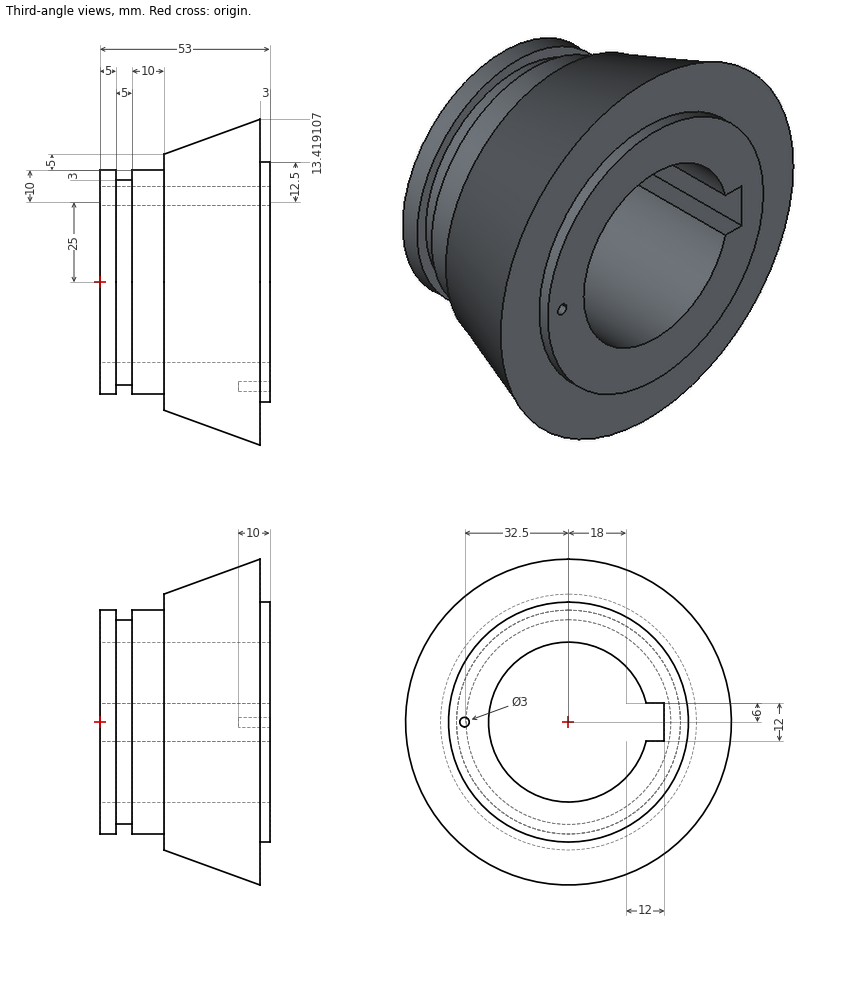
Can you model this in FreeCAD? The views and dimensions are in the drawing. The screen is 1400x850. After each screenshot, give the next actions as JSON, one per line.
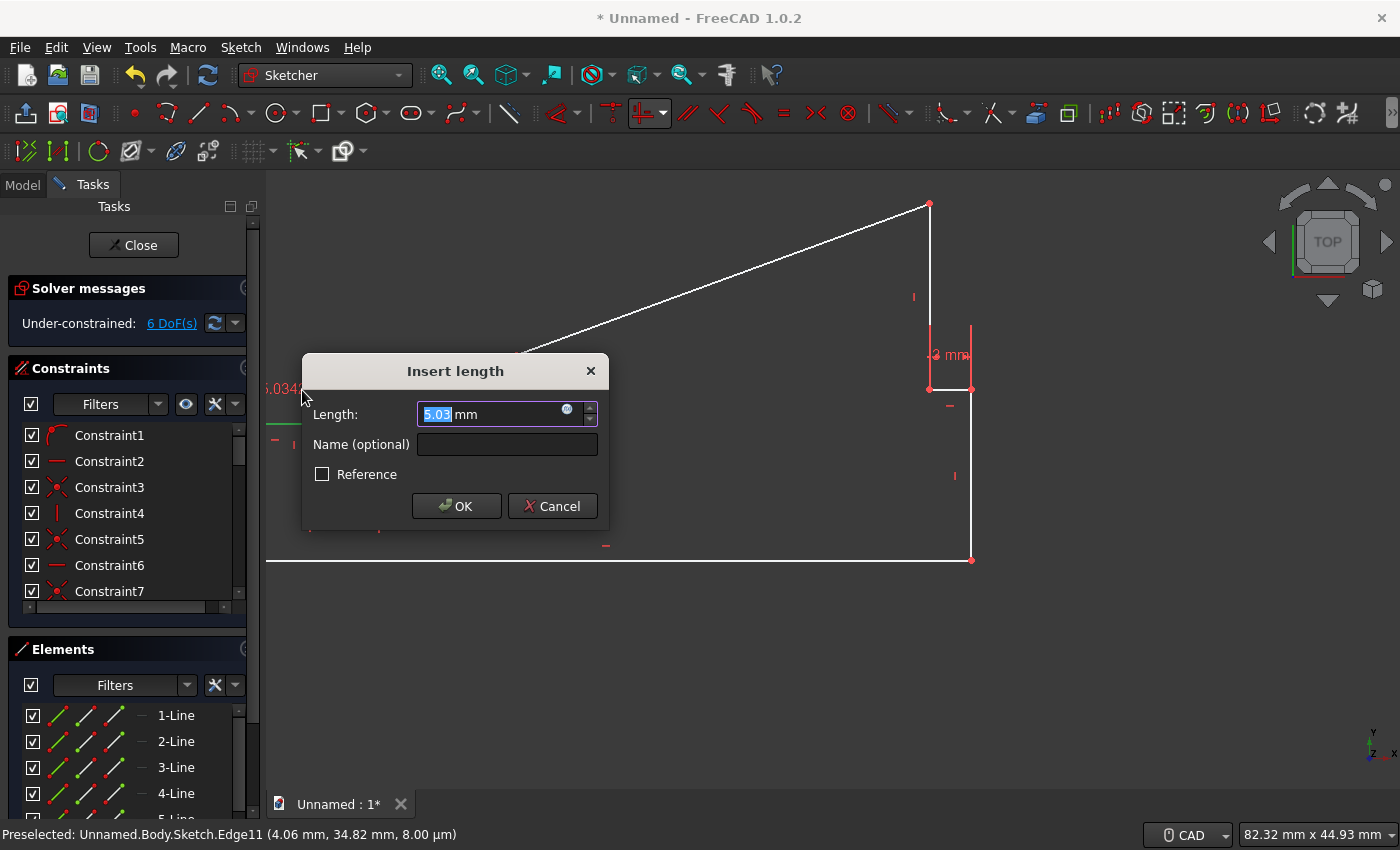
{"action": "type", "text": "5"}
{"action": "key", "text": "Return"}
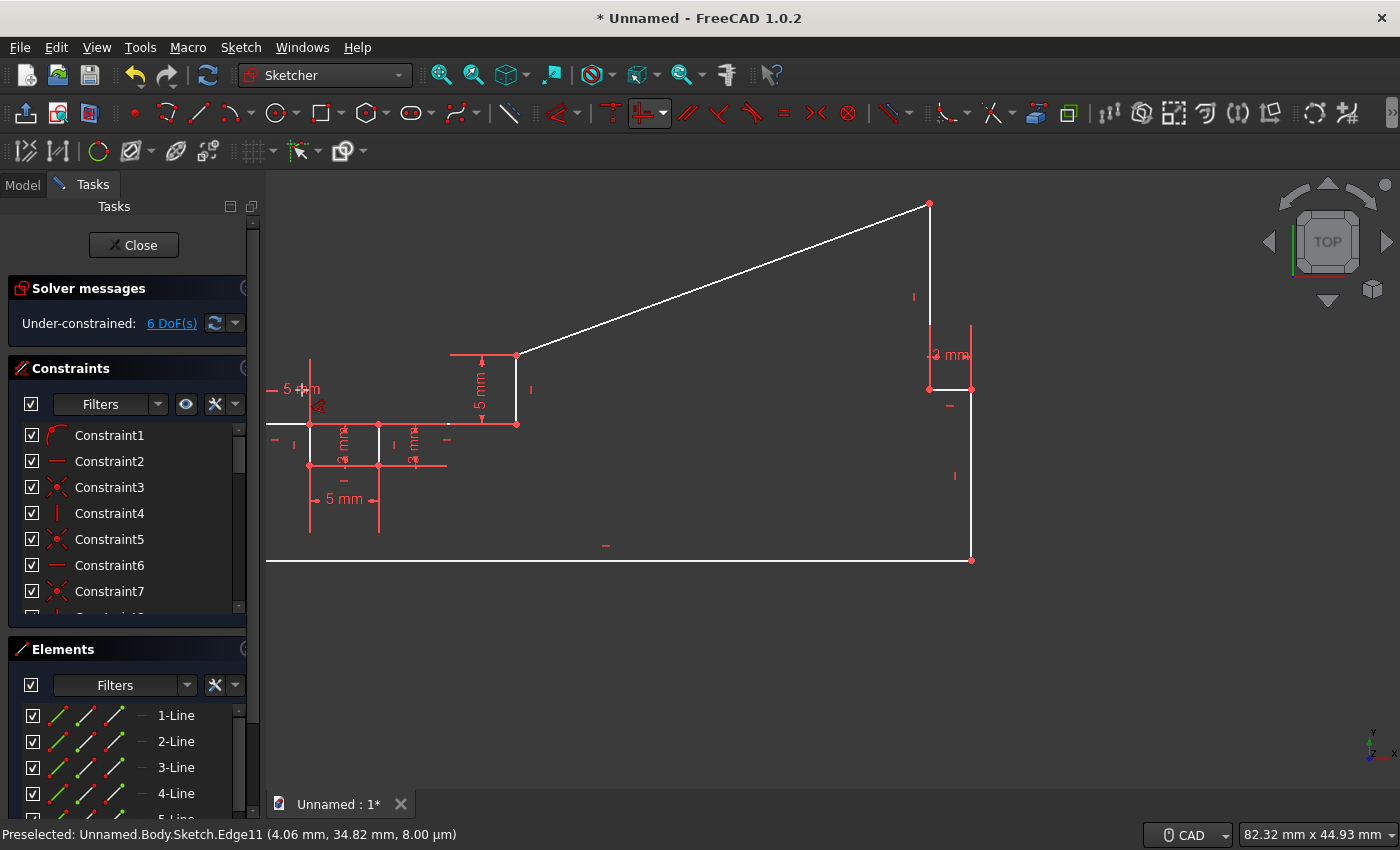
{"action": "left_click", "coordinate": [460, 561]}
{"action": "left_click", "coordinate": [633, 595]}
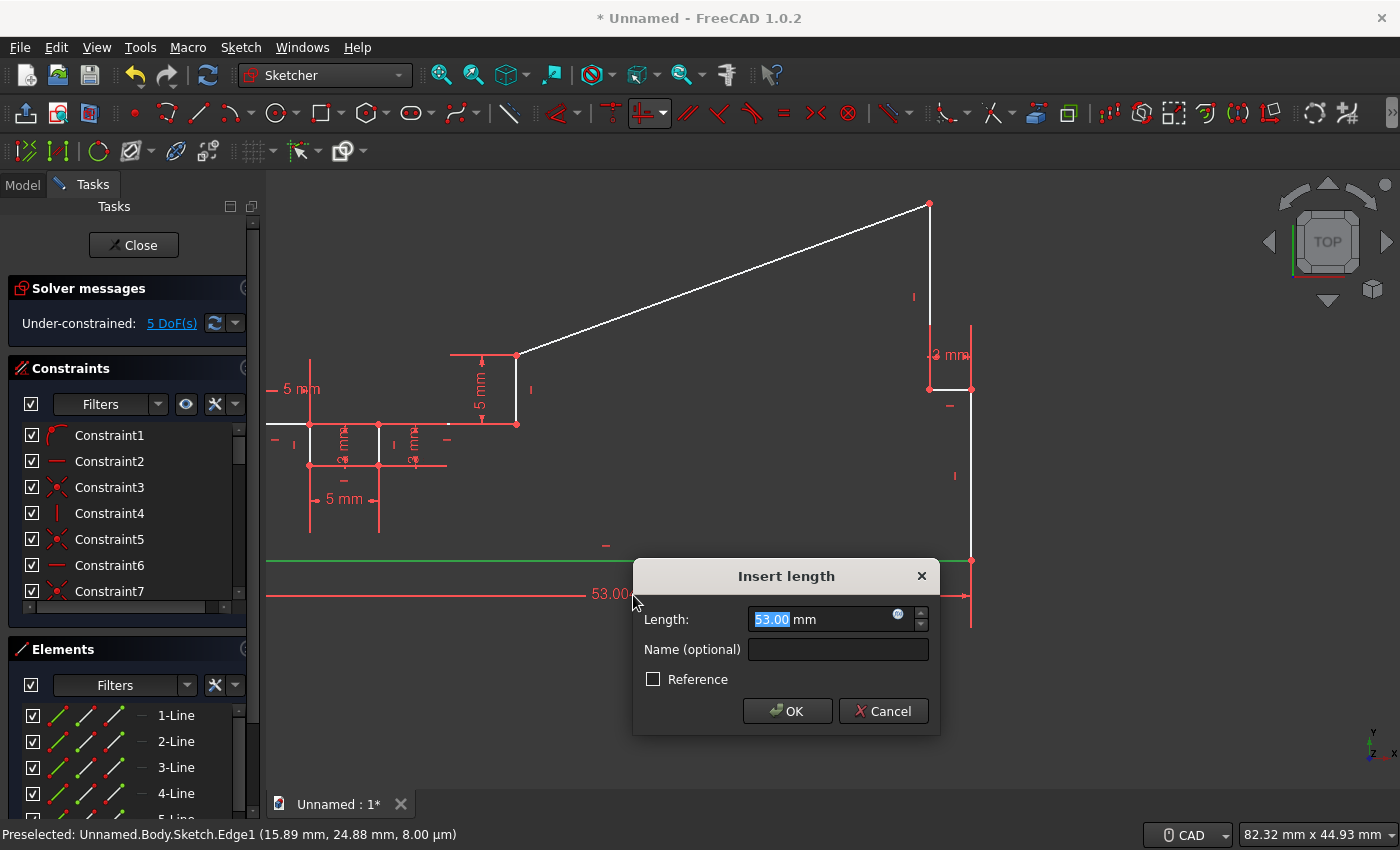
{"action": "type", "text": "53"}
{"action": "key", "text": "Return"}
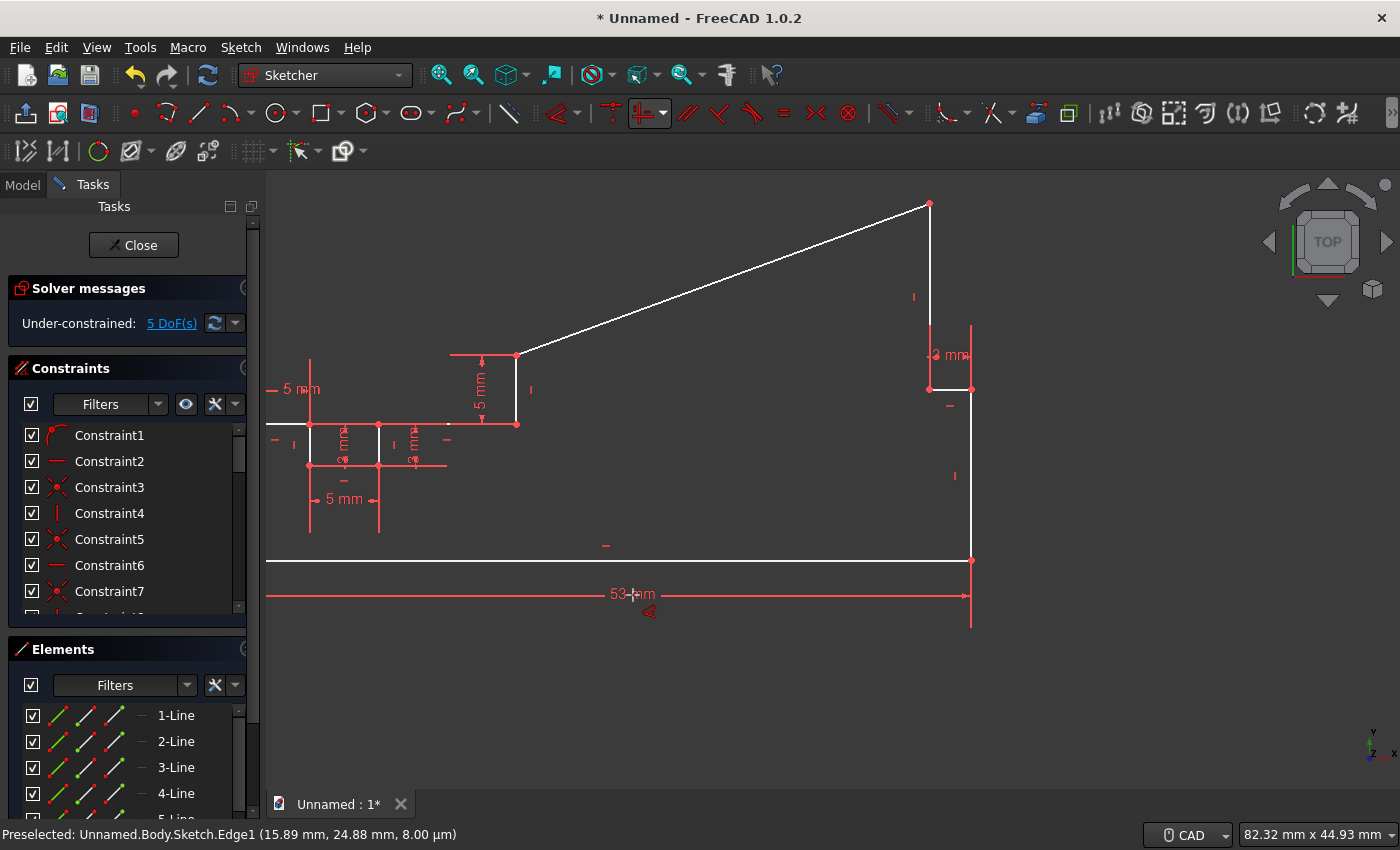
{"action": "left_click", "coordinate": [475, 424]}
{"action": "left_click", "coordinate": [400, 390]}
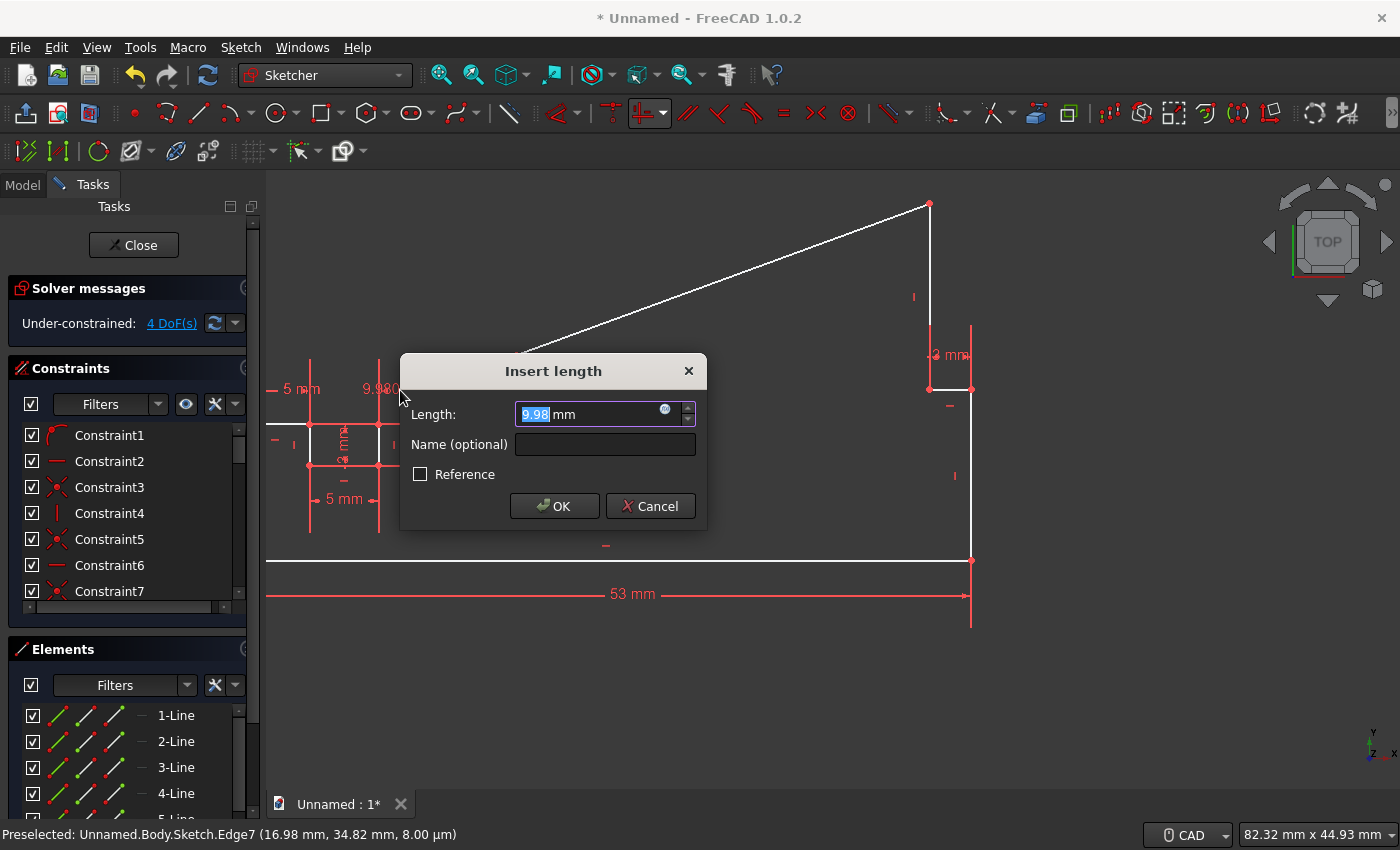
{"action": "type", "text": "10"}
{"action": "key", "text": "Return"}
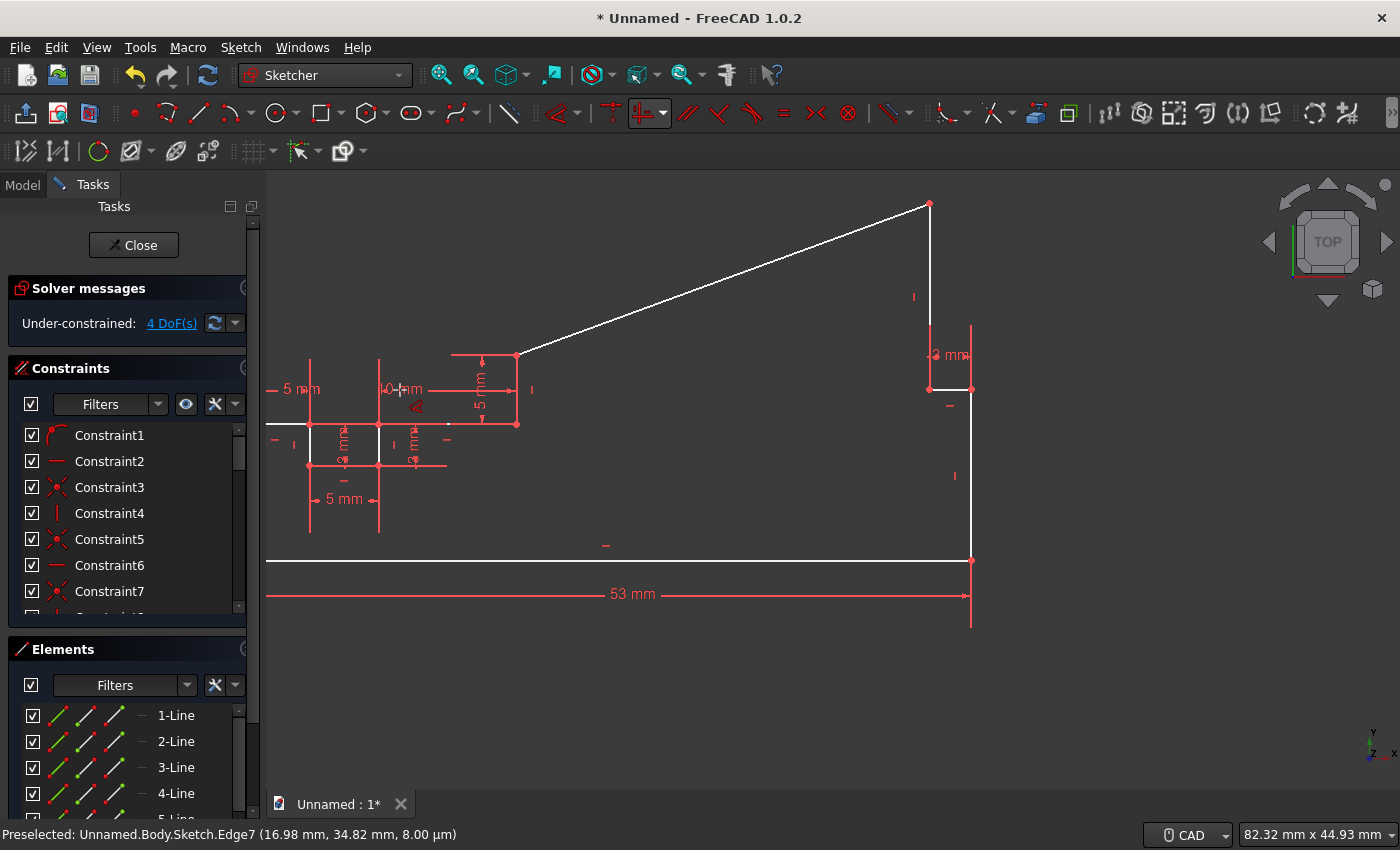
{"action": "scroll", "coordinate": [957, 390], "scroll_direction": "down", "scroll_amount": 3}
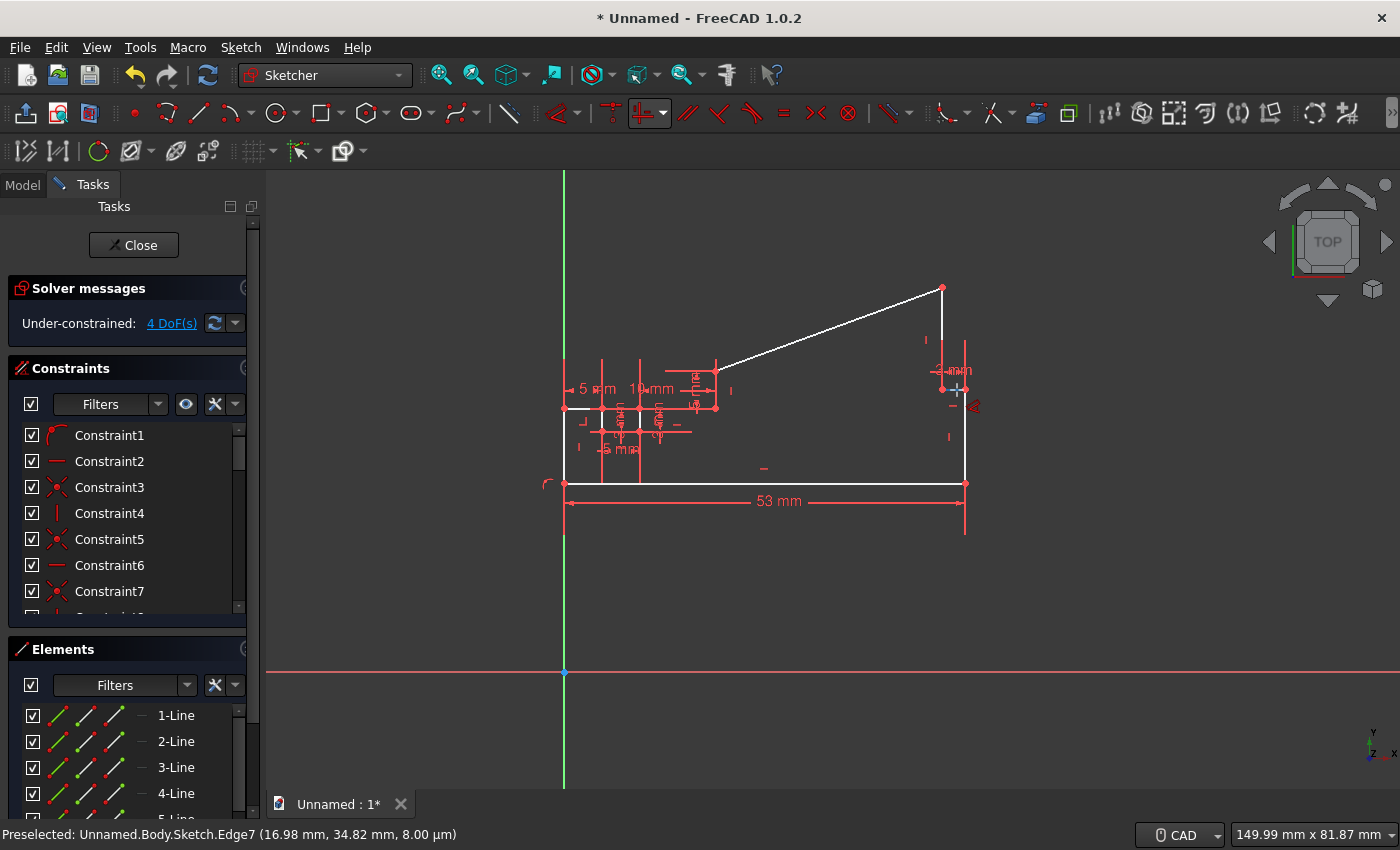
{"action": "left_click", "coordinate": [564, 431]}
{"action": "left_click", "coordinate": [530, 446]}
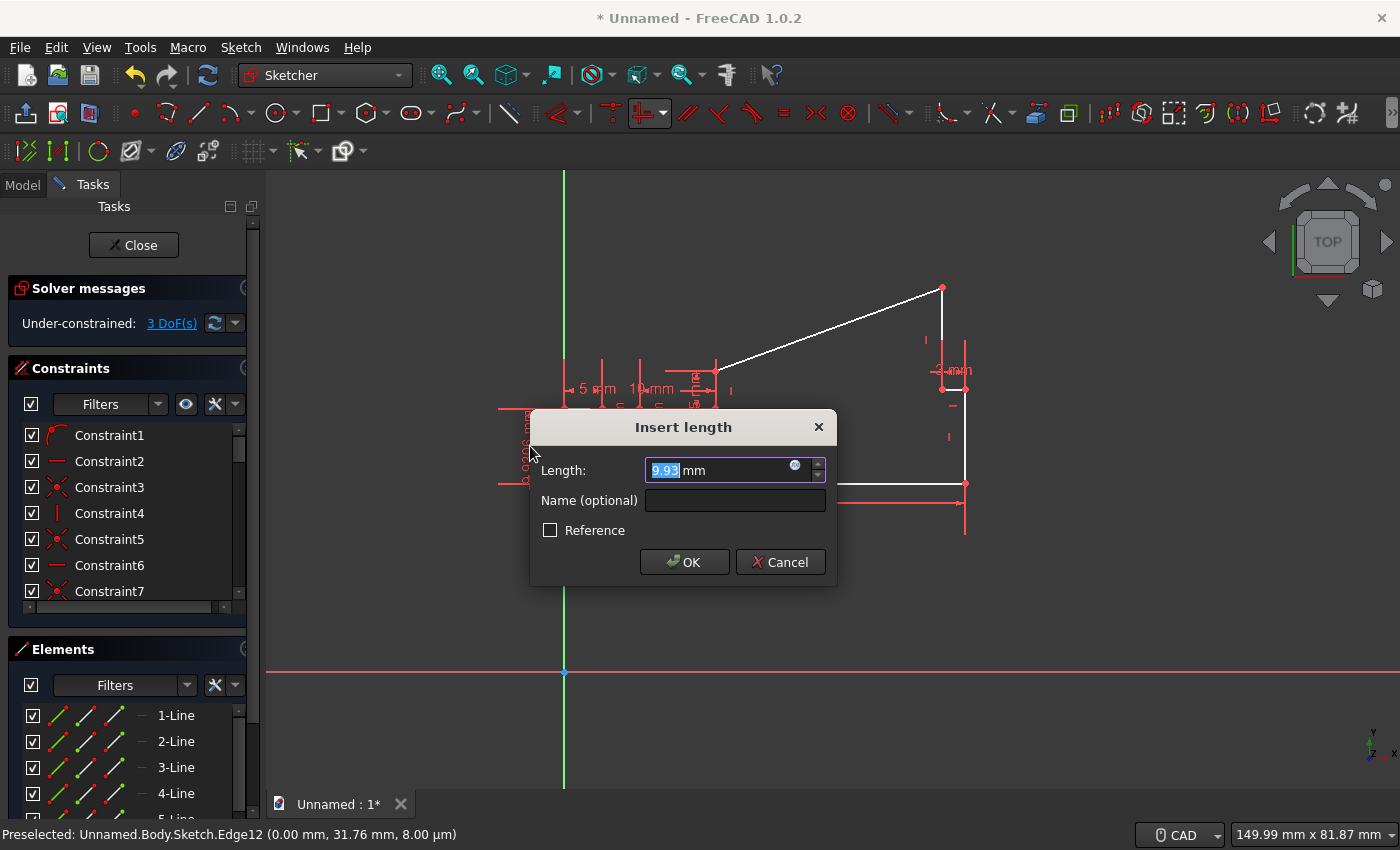
{"action": "type", "text": "10"}
{"action": "key", "text": "Return"}